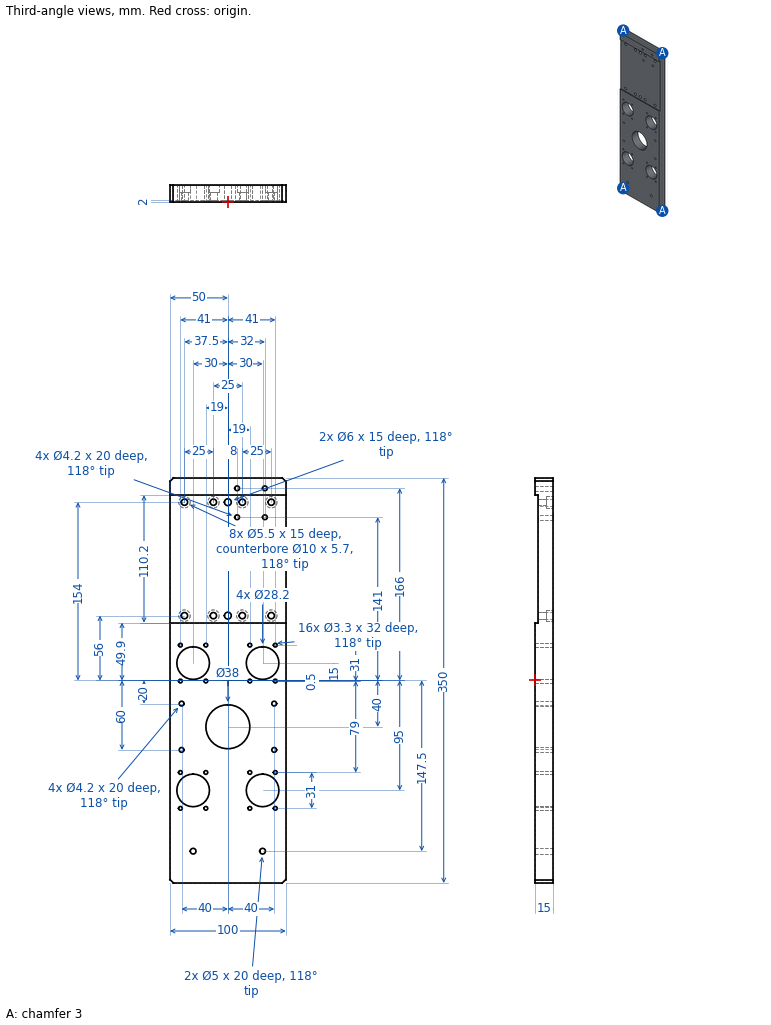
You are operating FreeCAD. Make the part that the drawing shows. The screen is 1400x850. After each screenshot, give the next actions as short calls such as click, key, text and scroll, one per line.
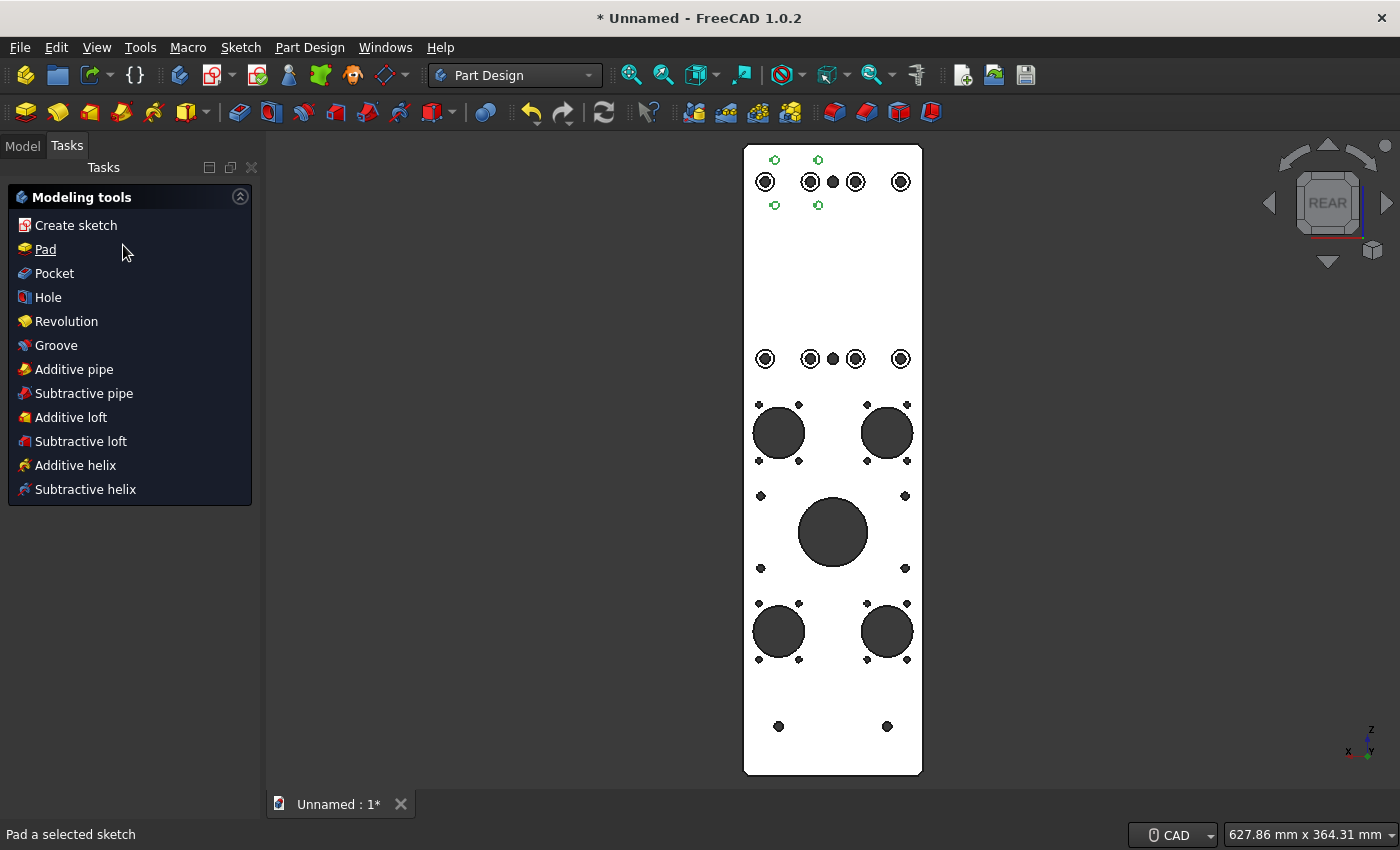
click(272, 112)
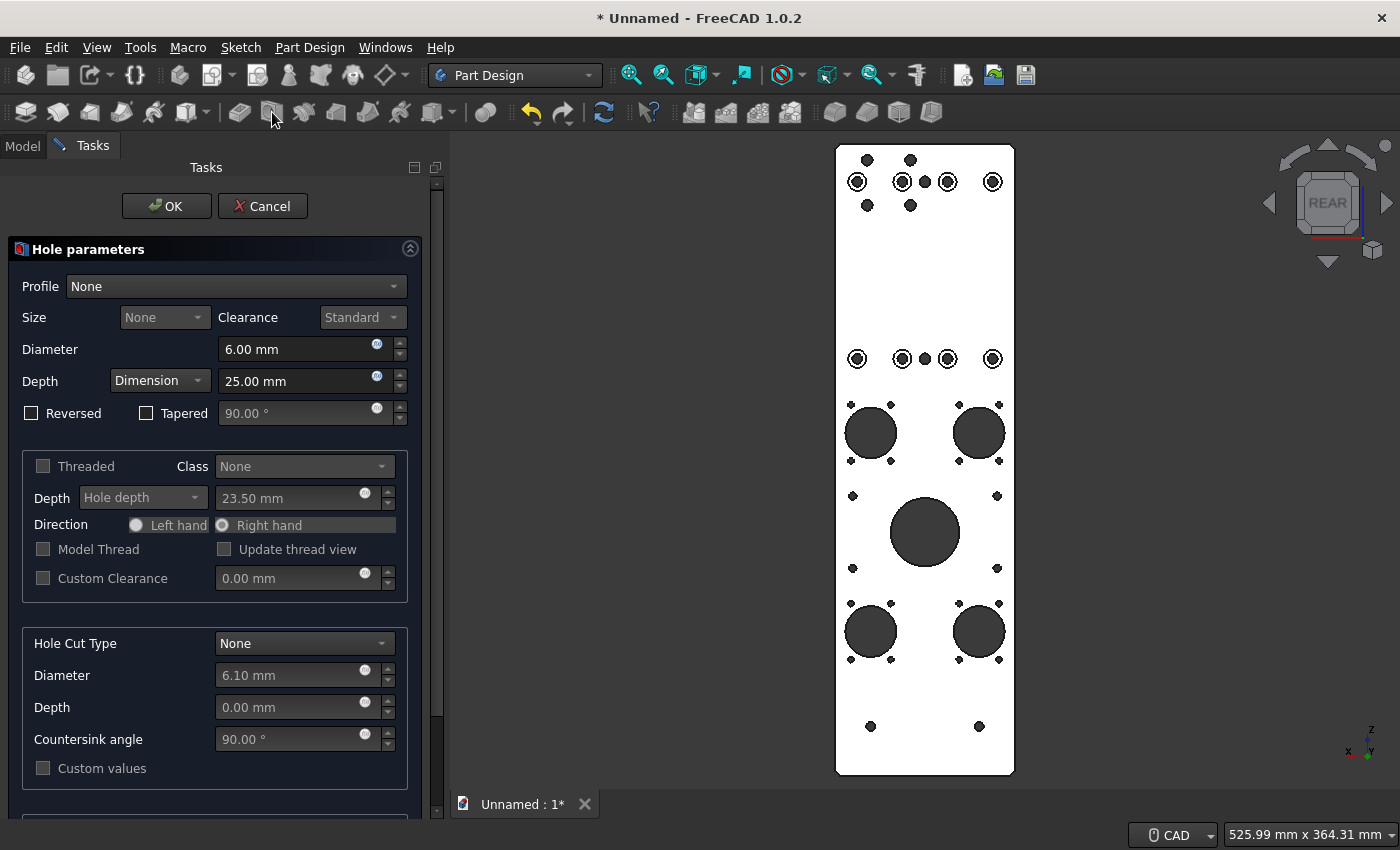
triple_click(305, 349)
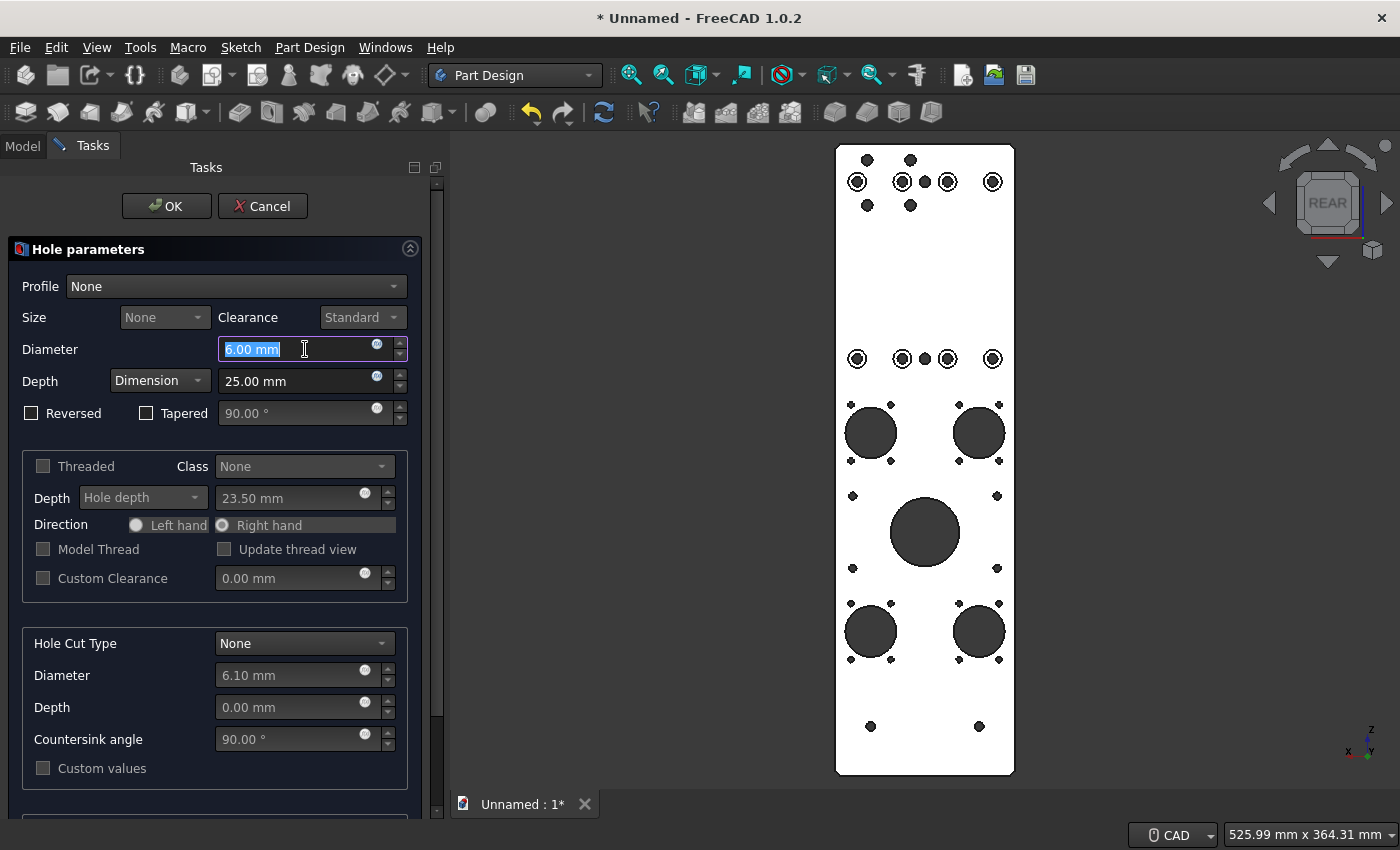
text(4.2)
key(Tab)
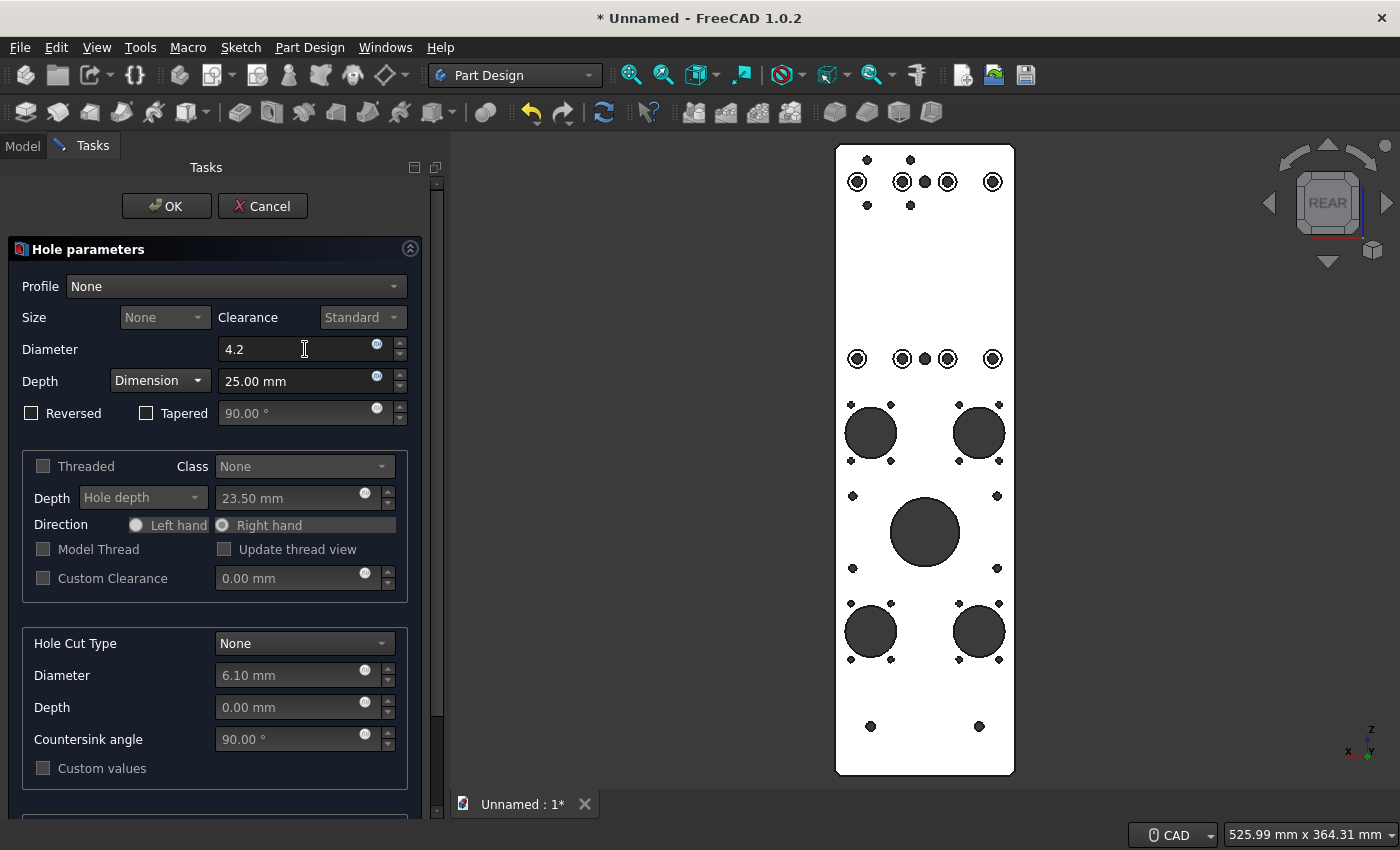
triple_click(305, 381)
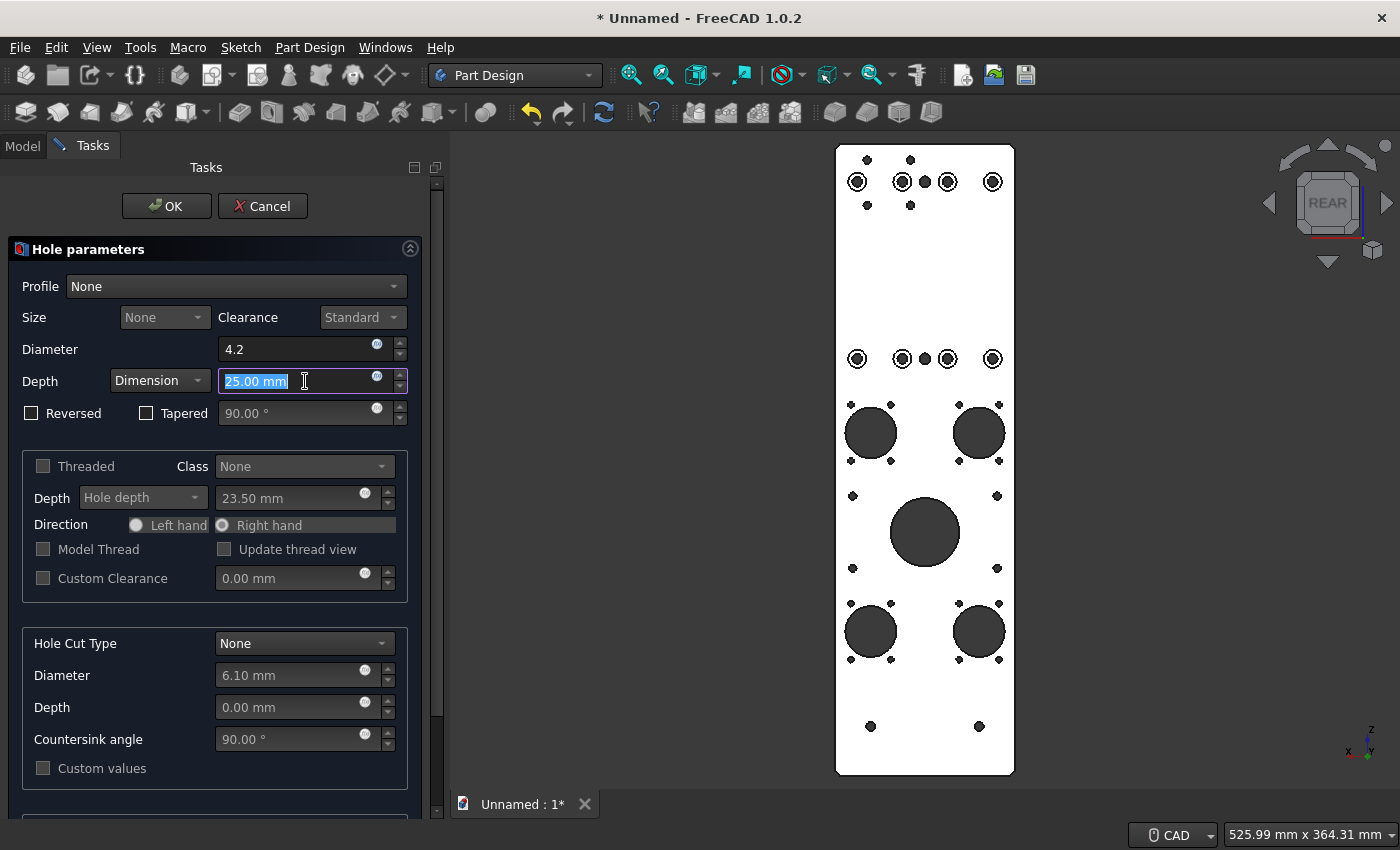
text(20)
key(Tab)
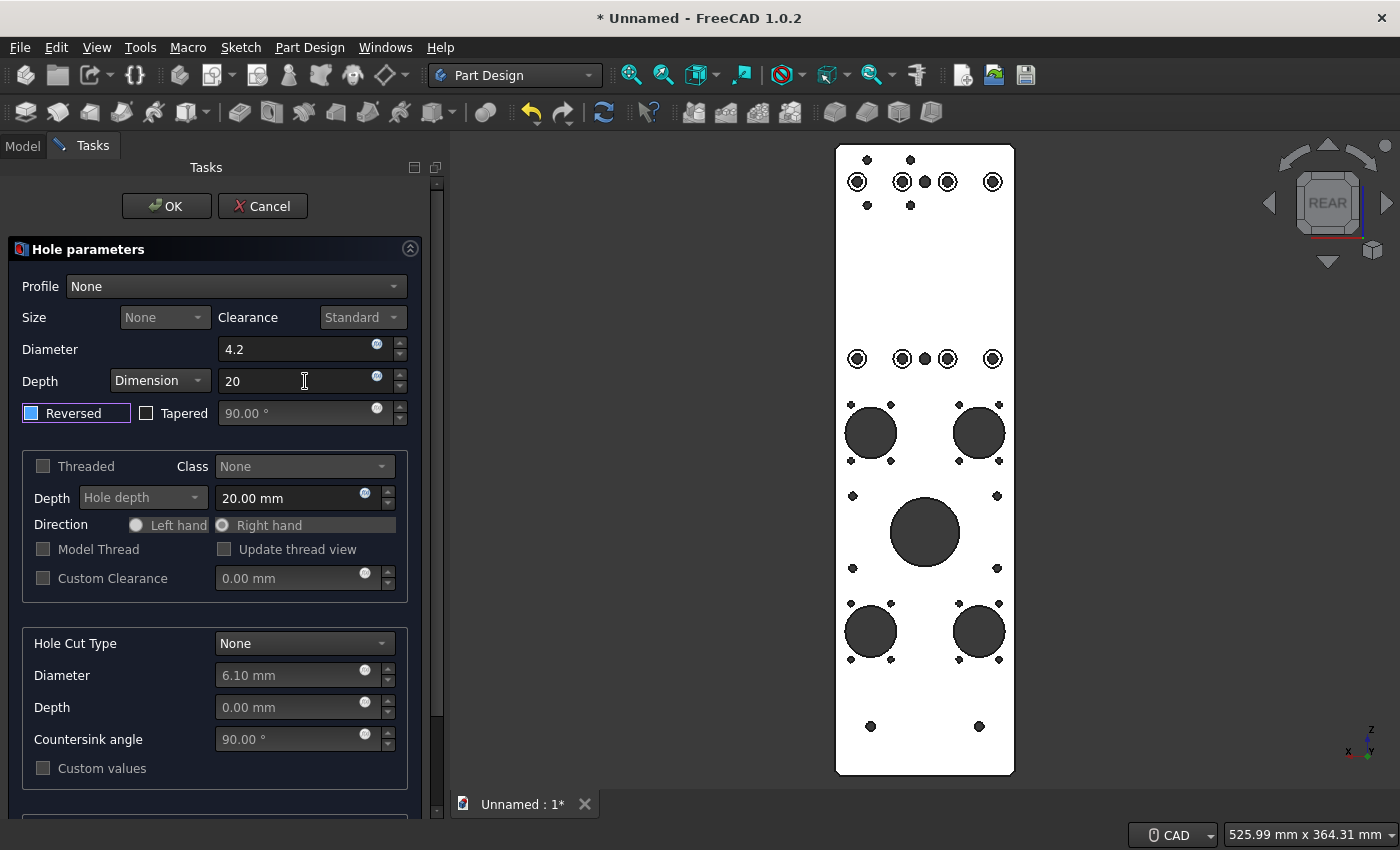
click(167, 206)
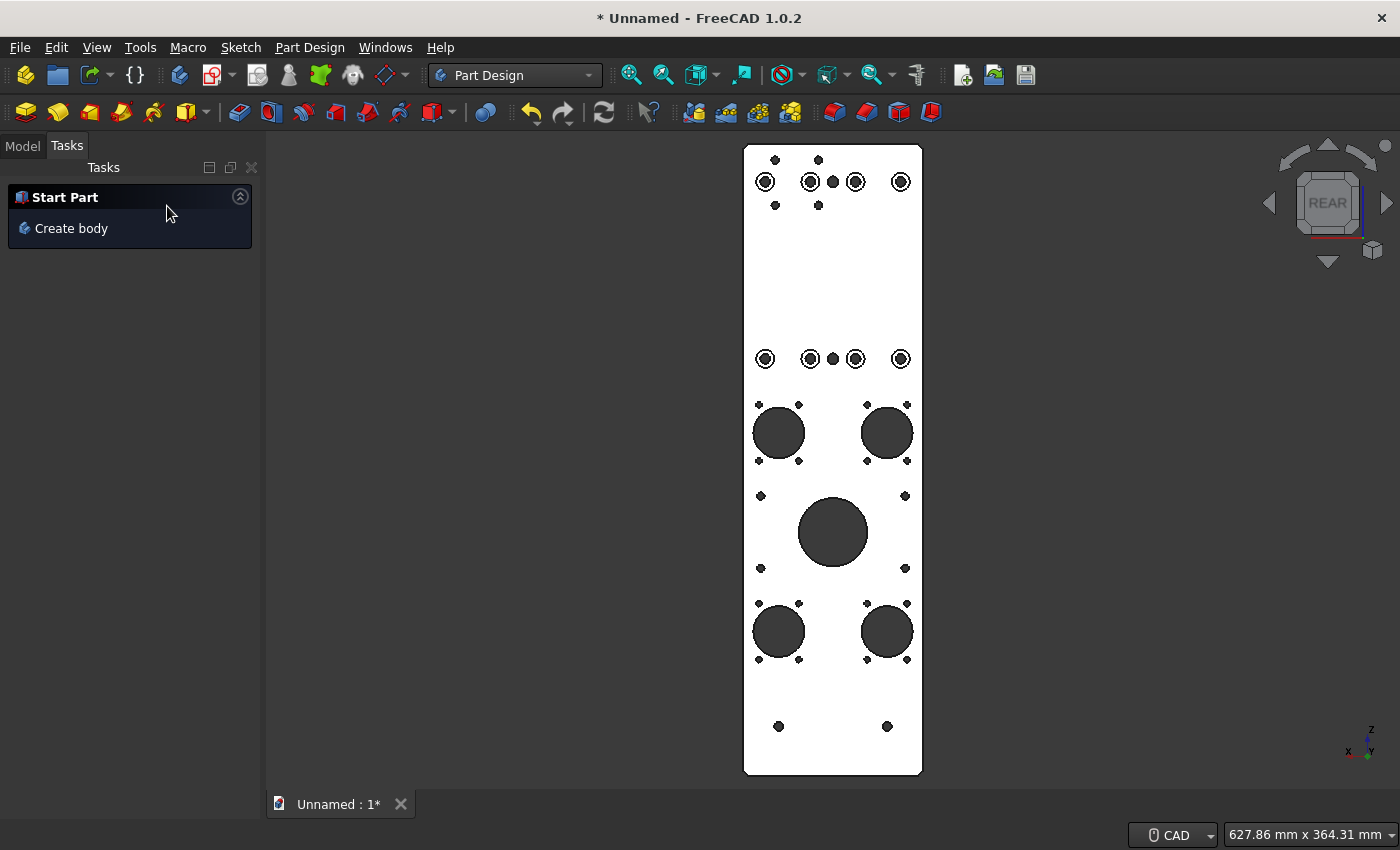
key(0)